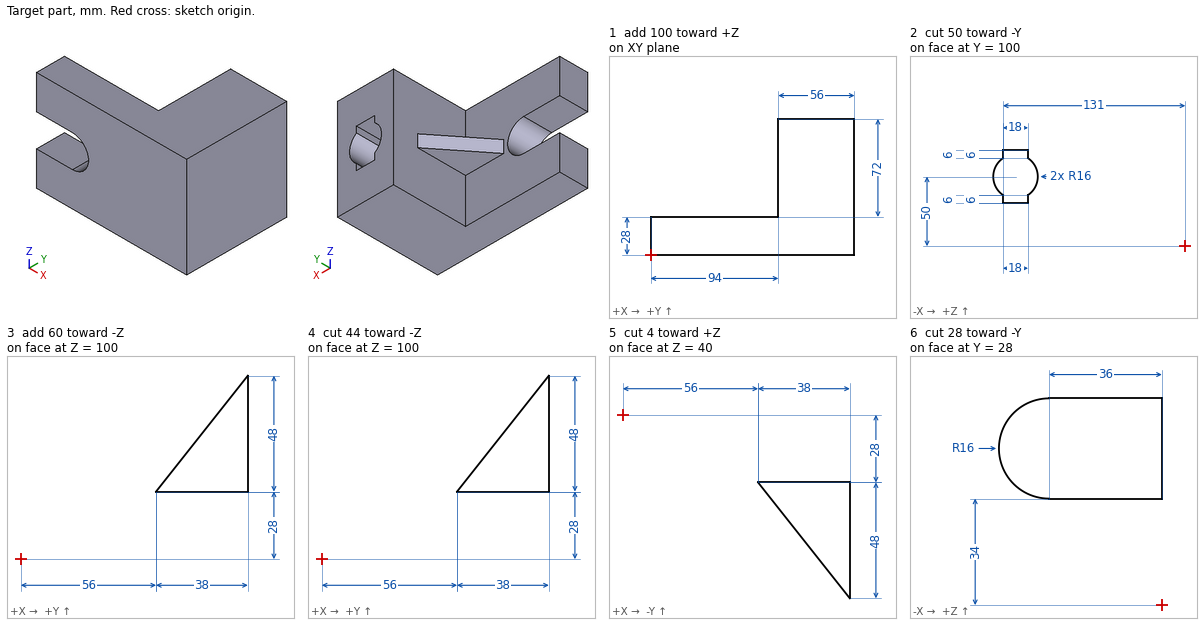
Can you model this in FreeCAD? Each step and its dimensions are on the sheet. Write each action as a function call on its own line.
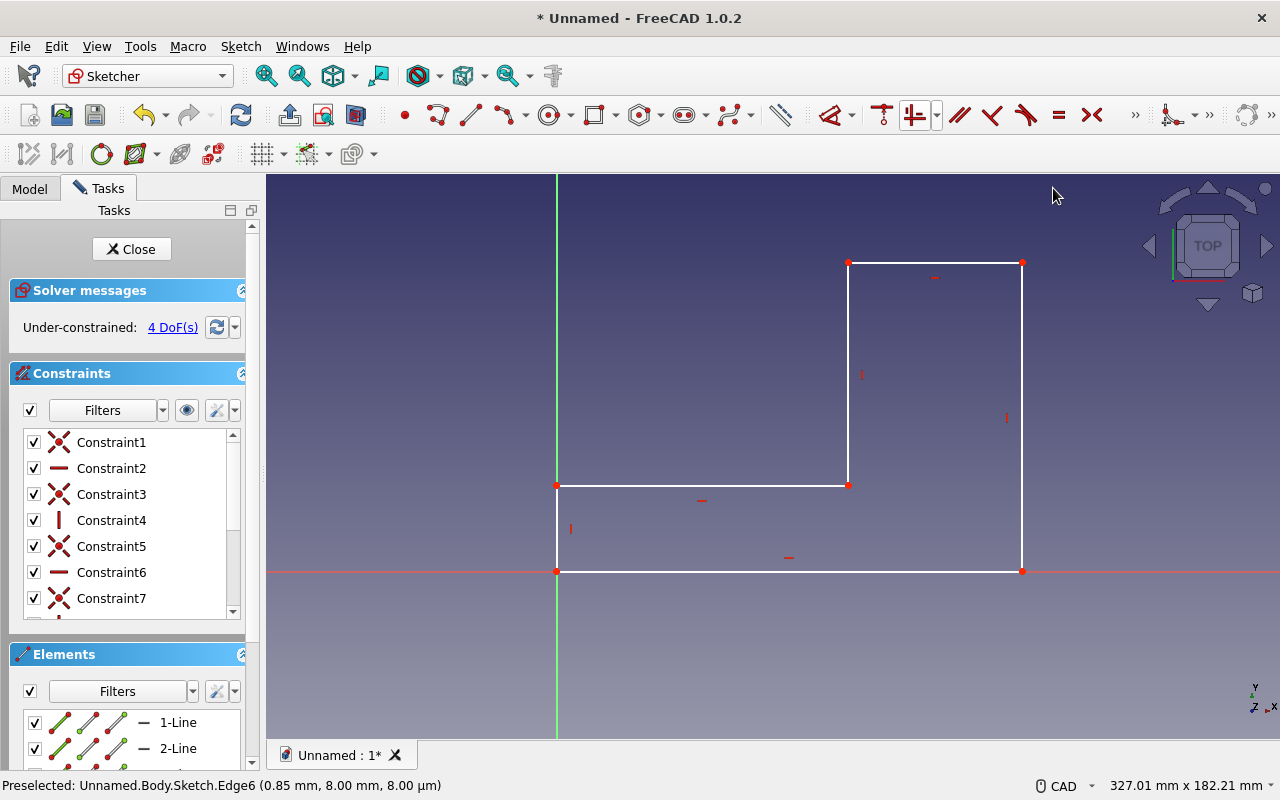
click(970, 263)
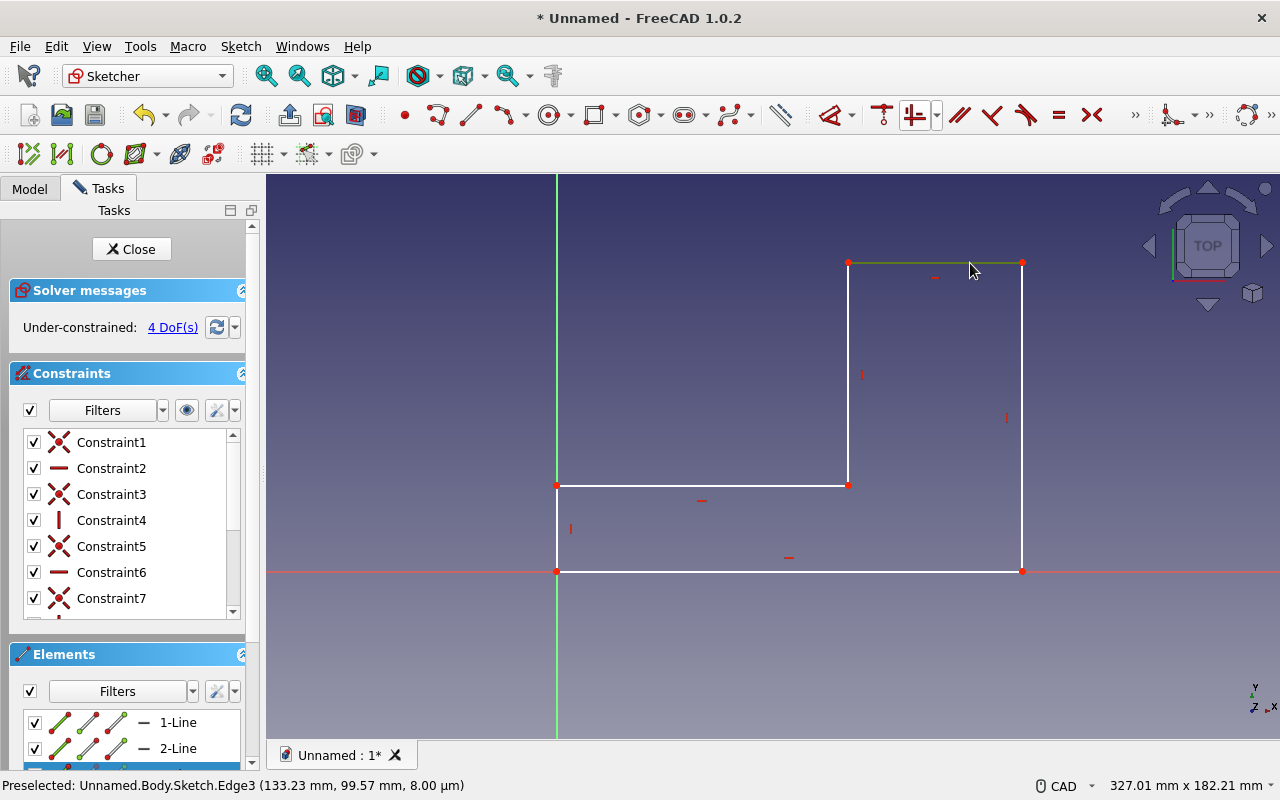
key(l)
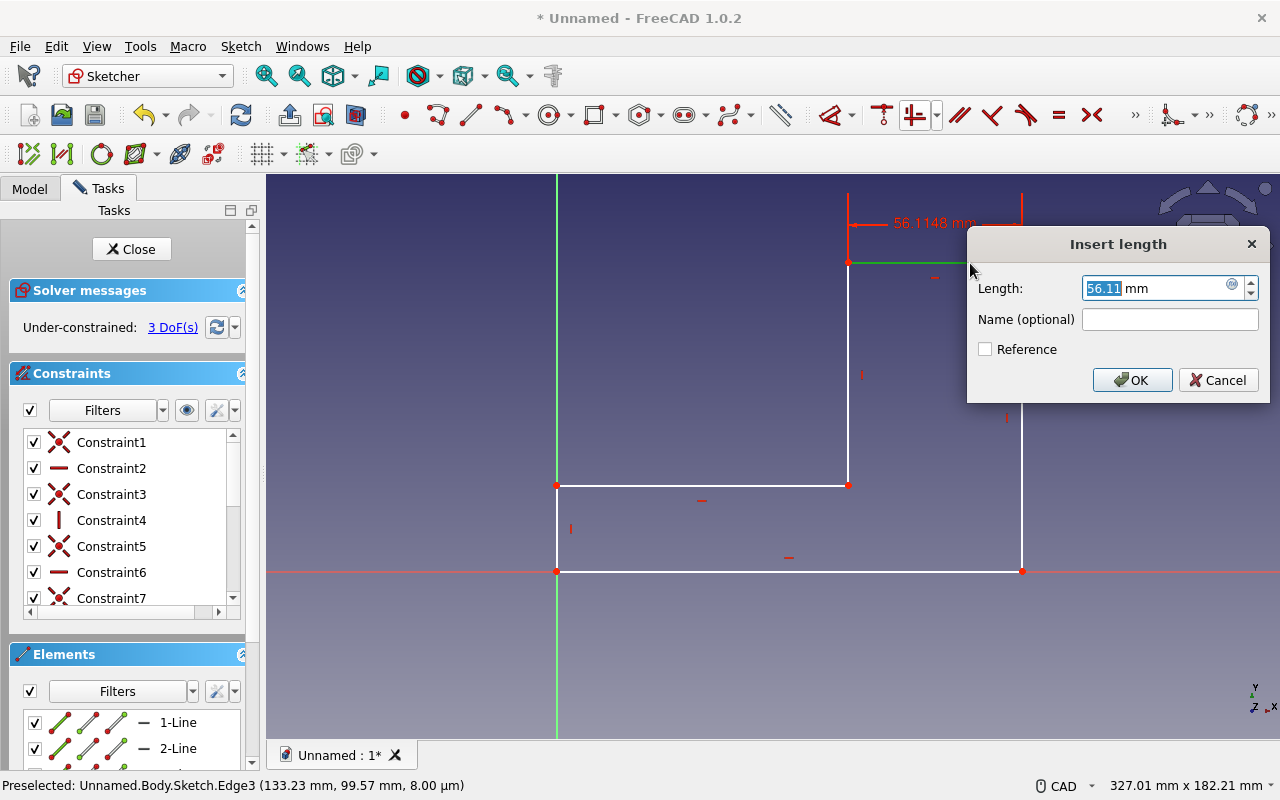
text(56)
key(Return)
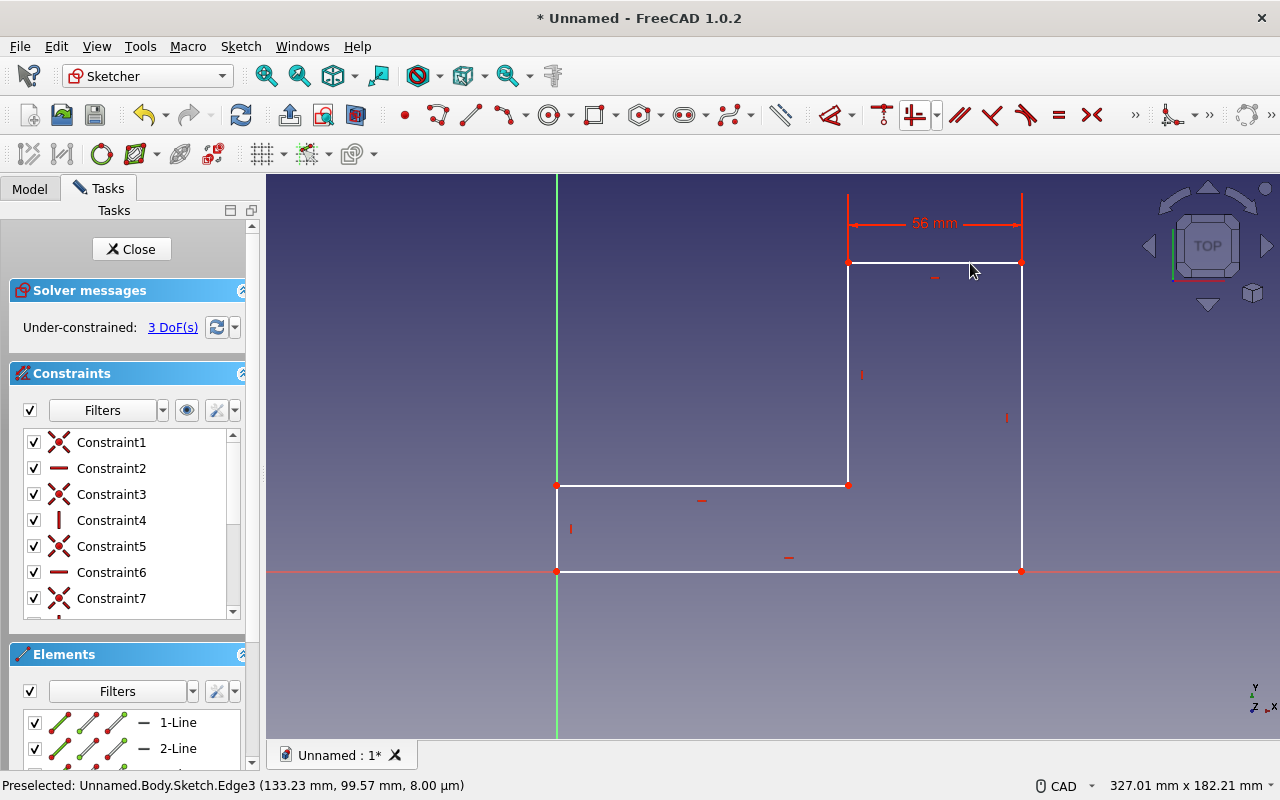
click(848, 330)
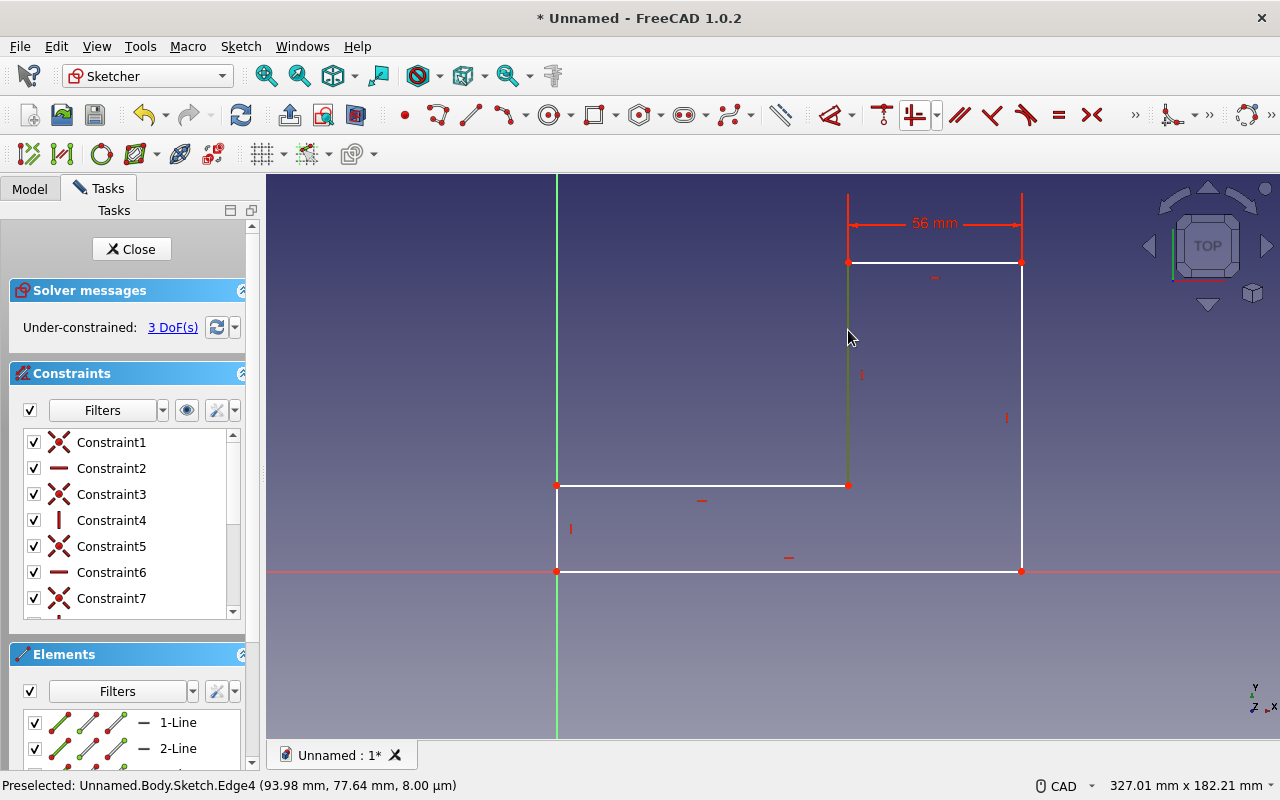
click(852, 116)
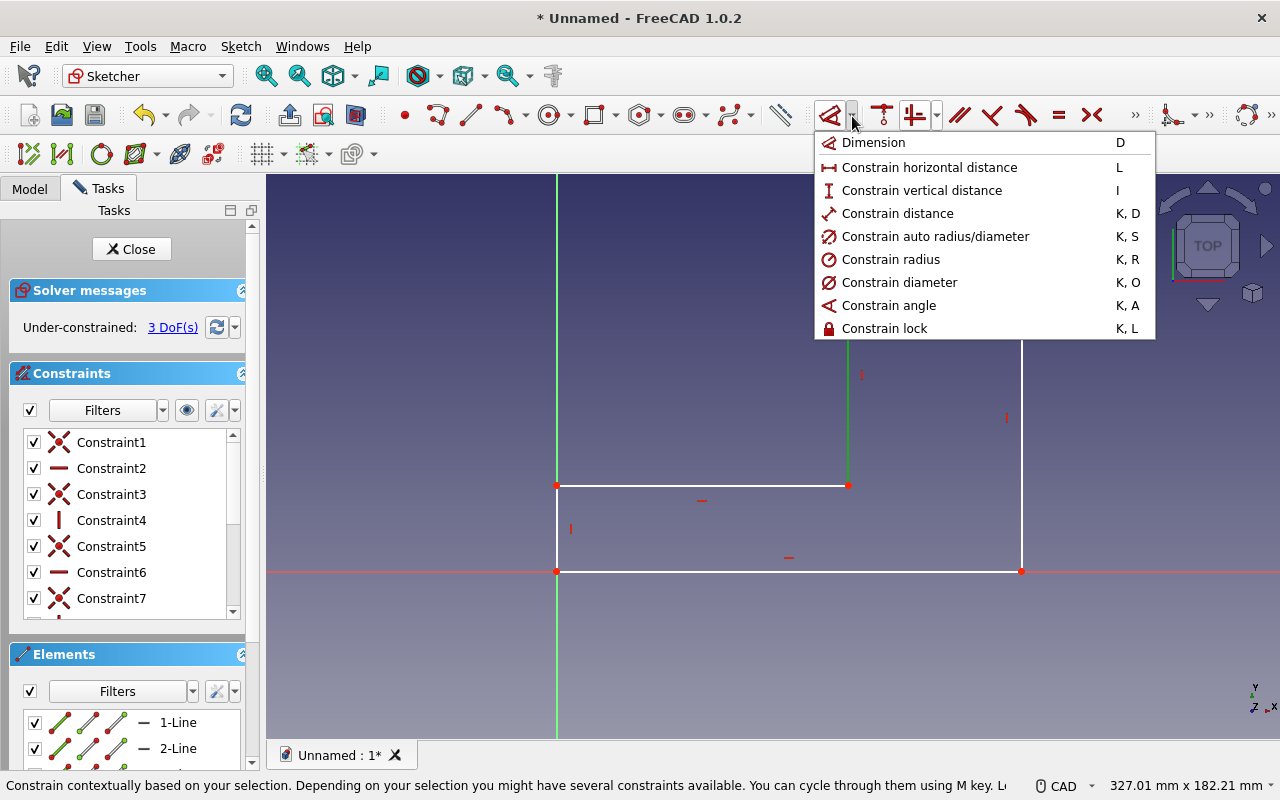
click(985, 190)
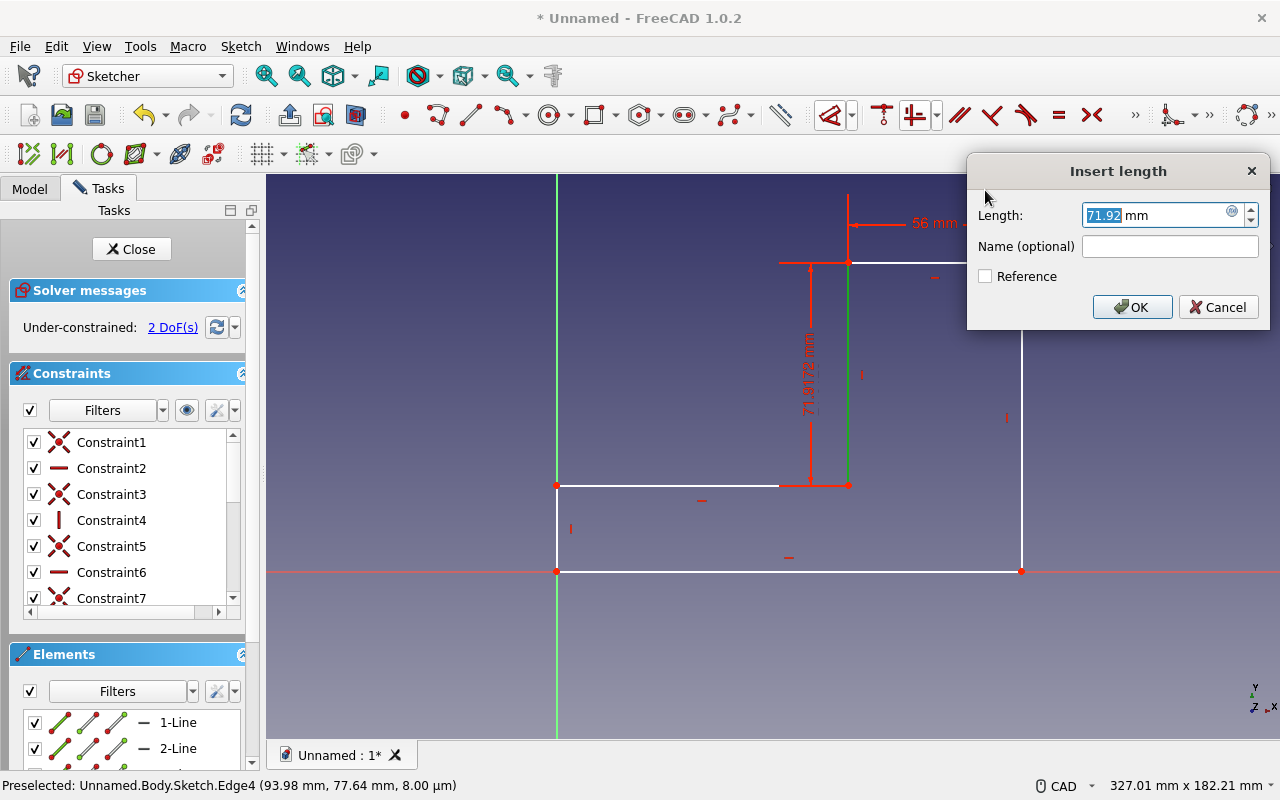
text(72)
key(Return)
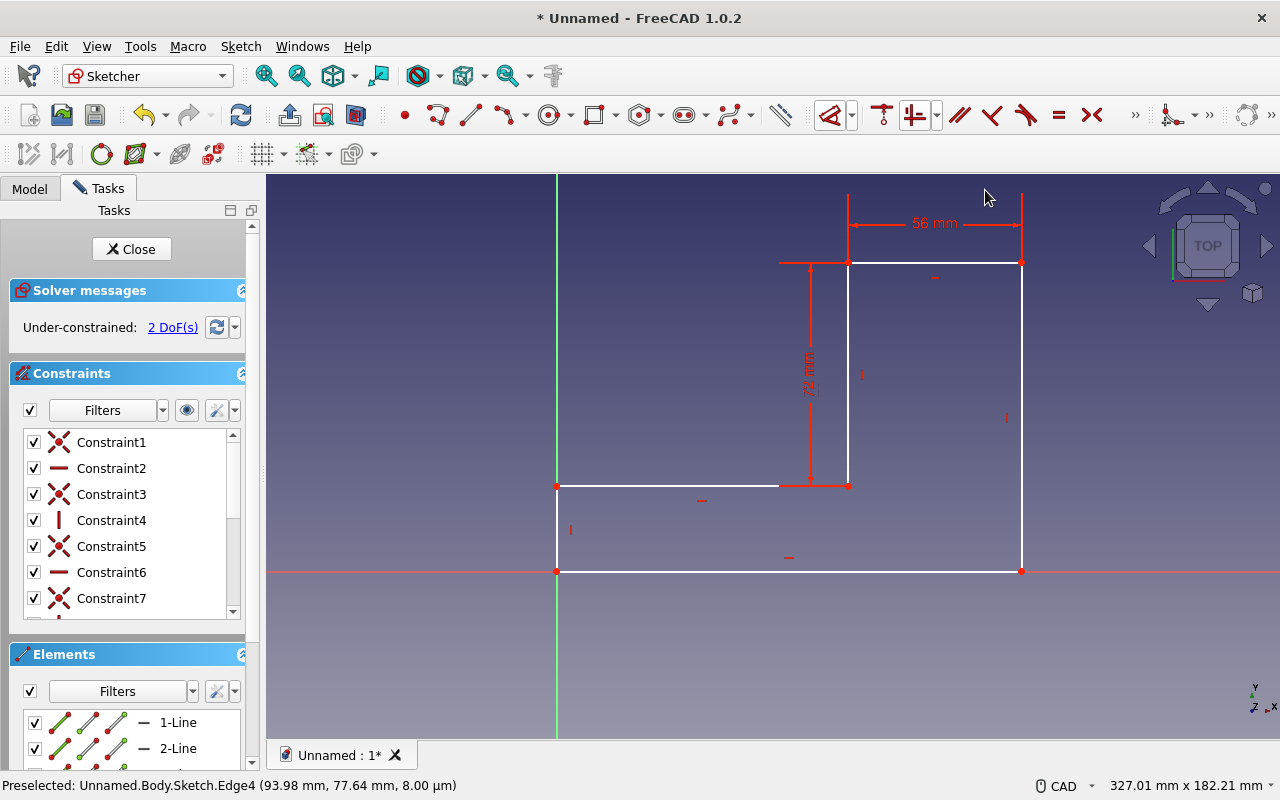
click(761, 486)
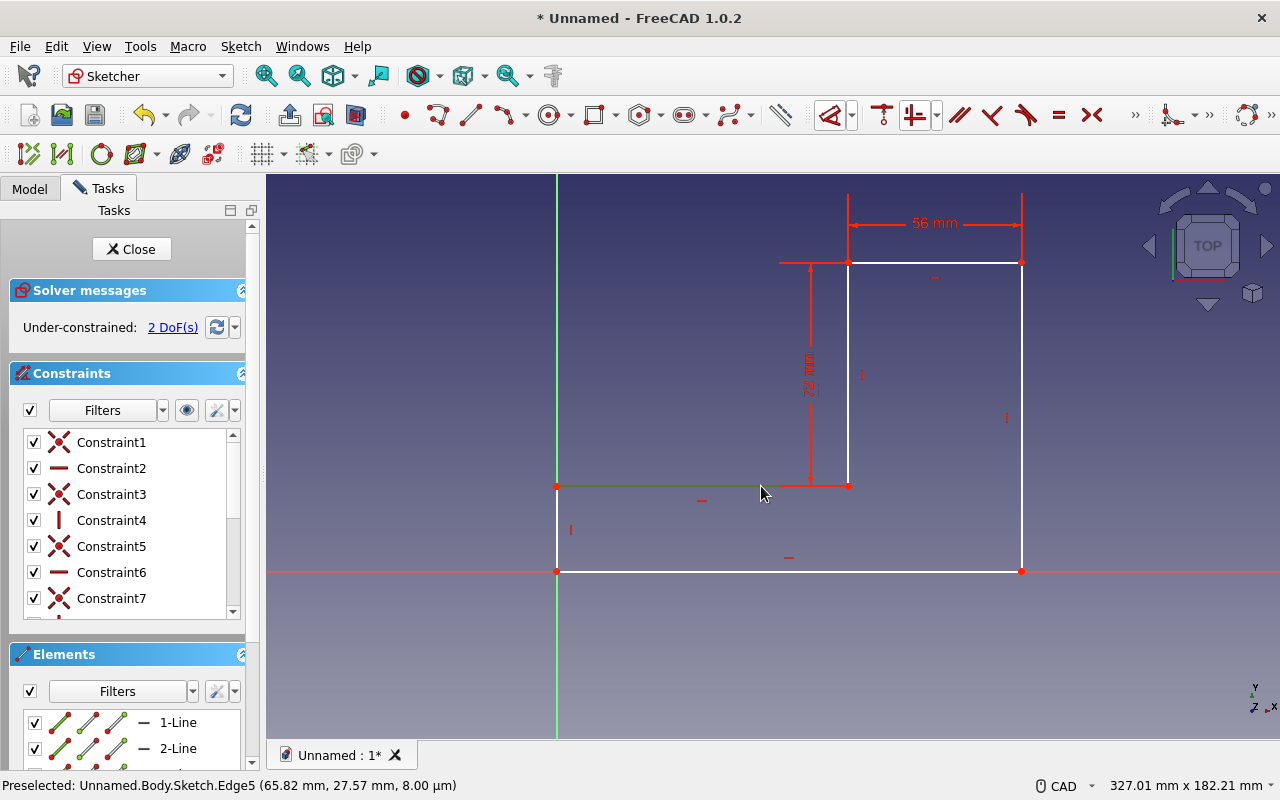
click(852, 116)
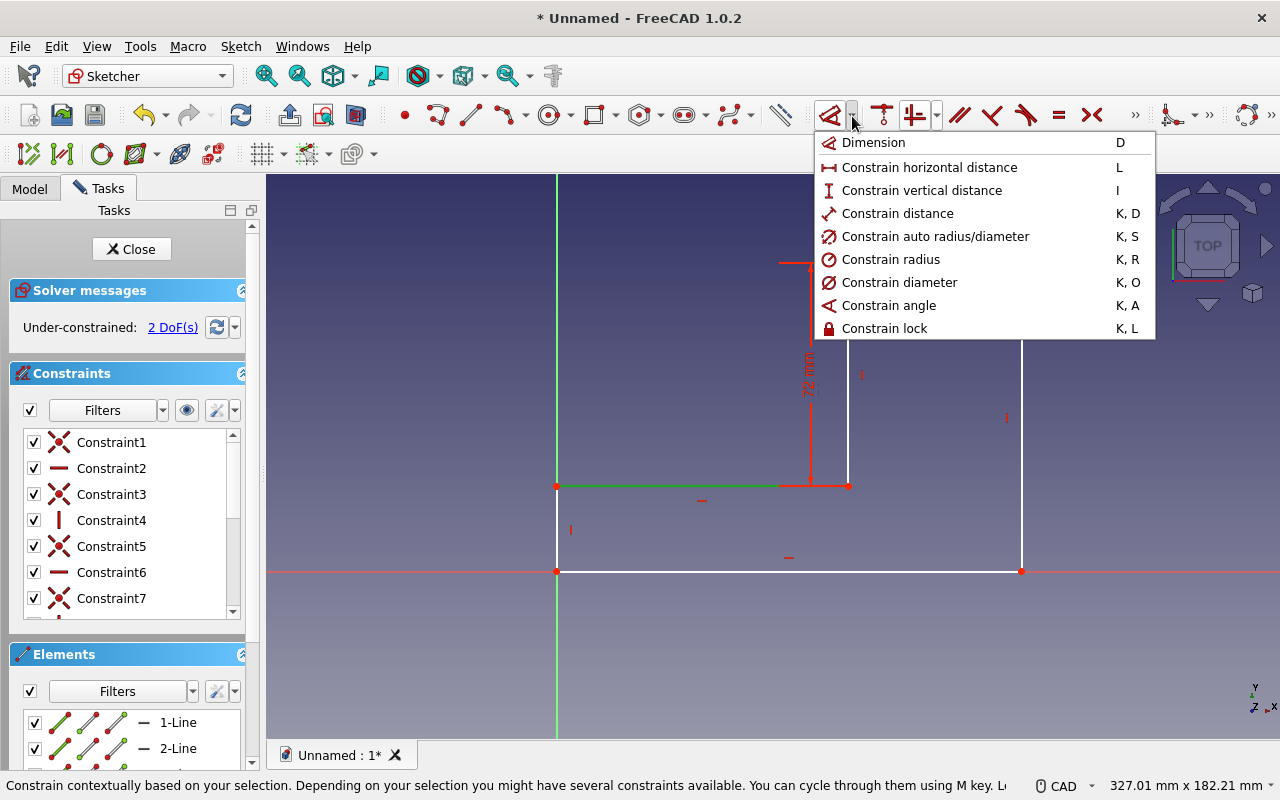
click(985, 168)